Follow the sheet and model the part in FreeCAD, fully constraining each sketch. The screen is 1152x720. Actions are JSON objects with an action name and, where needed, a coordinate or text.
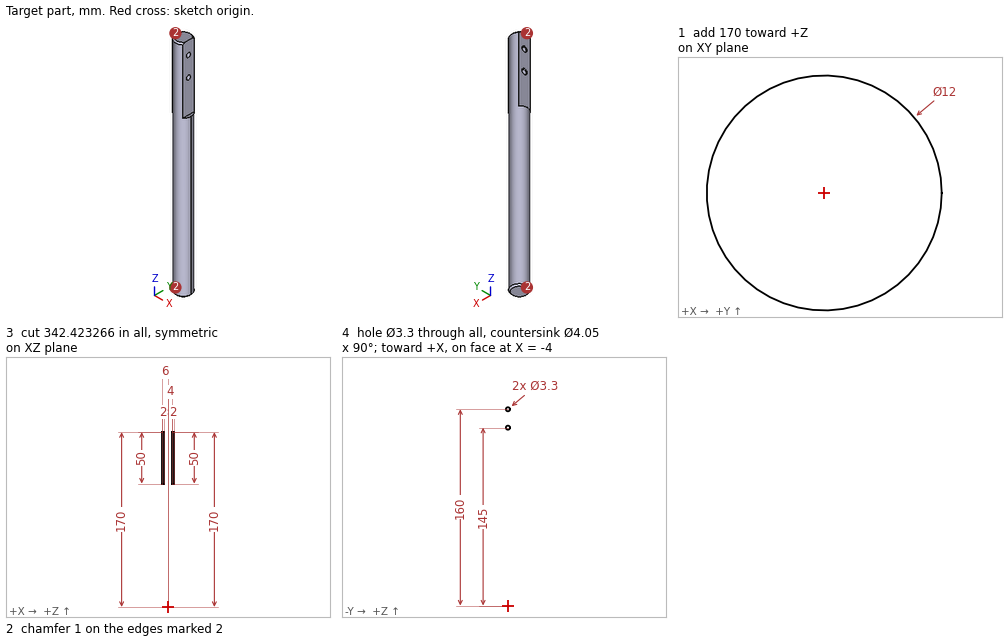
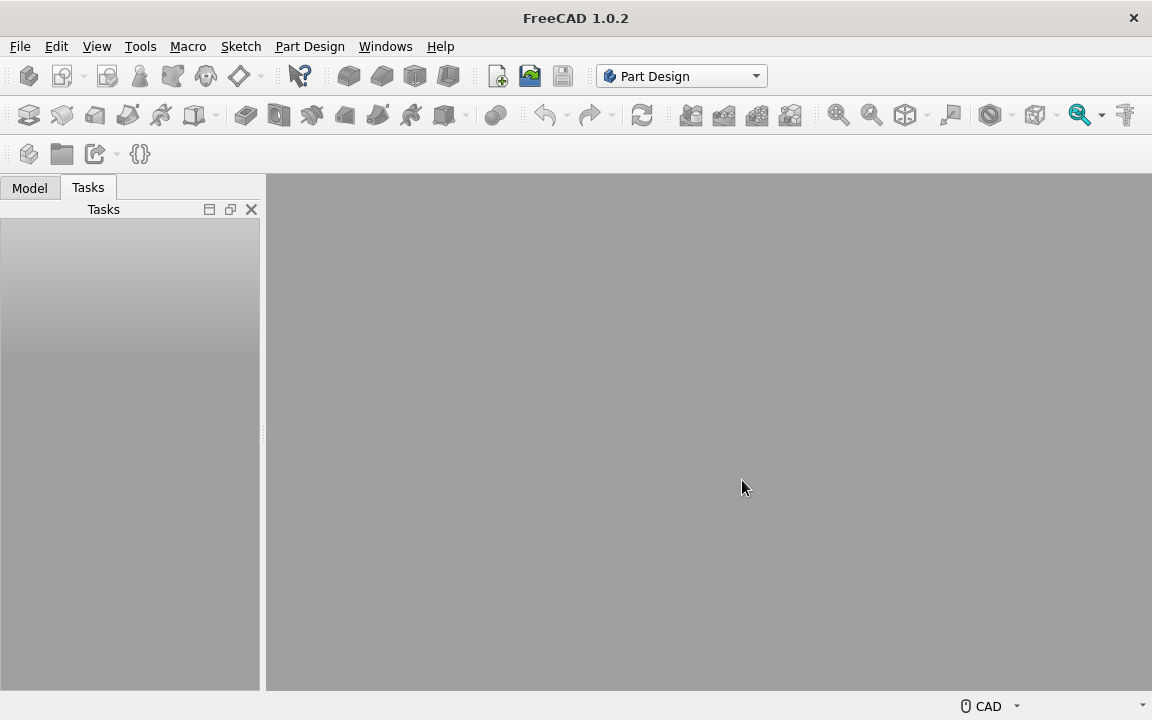
{"action": "key", "text": "ctrl+n"}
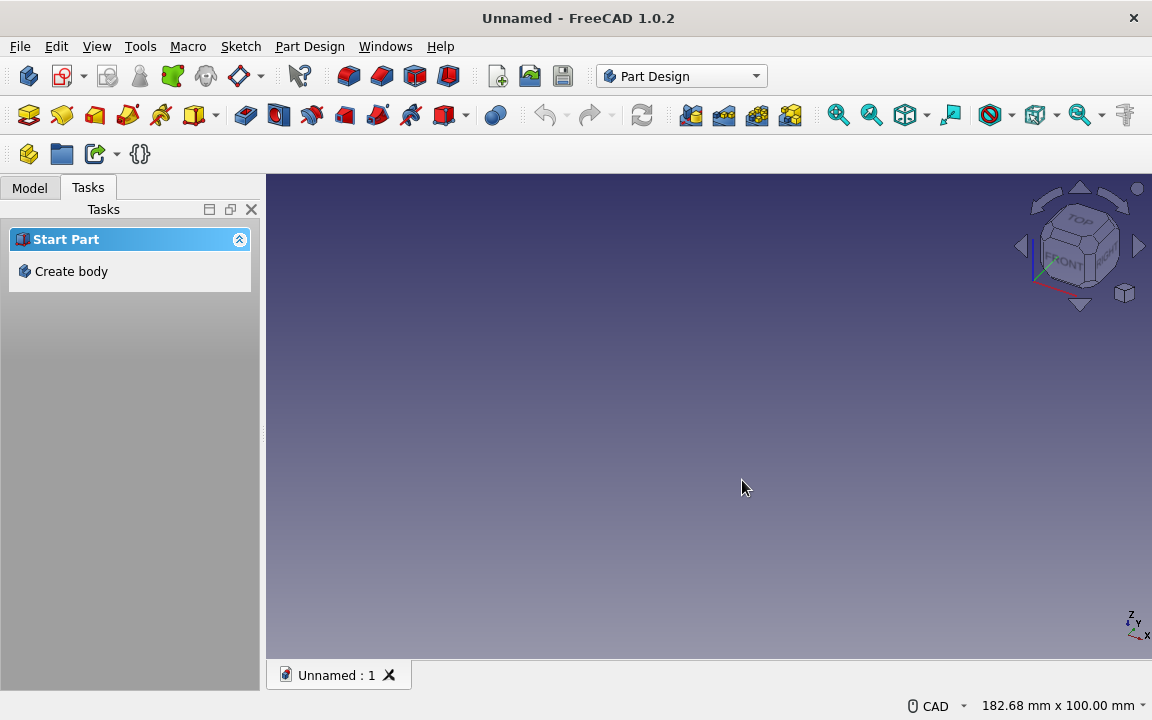
{"action": "left_click", "coordinate": [62, 76]}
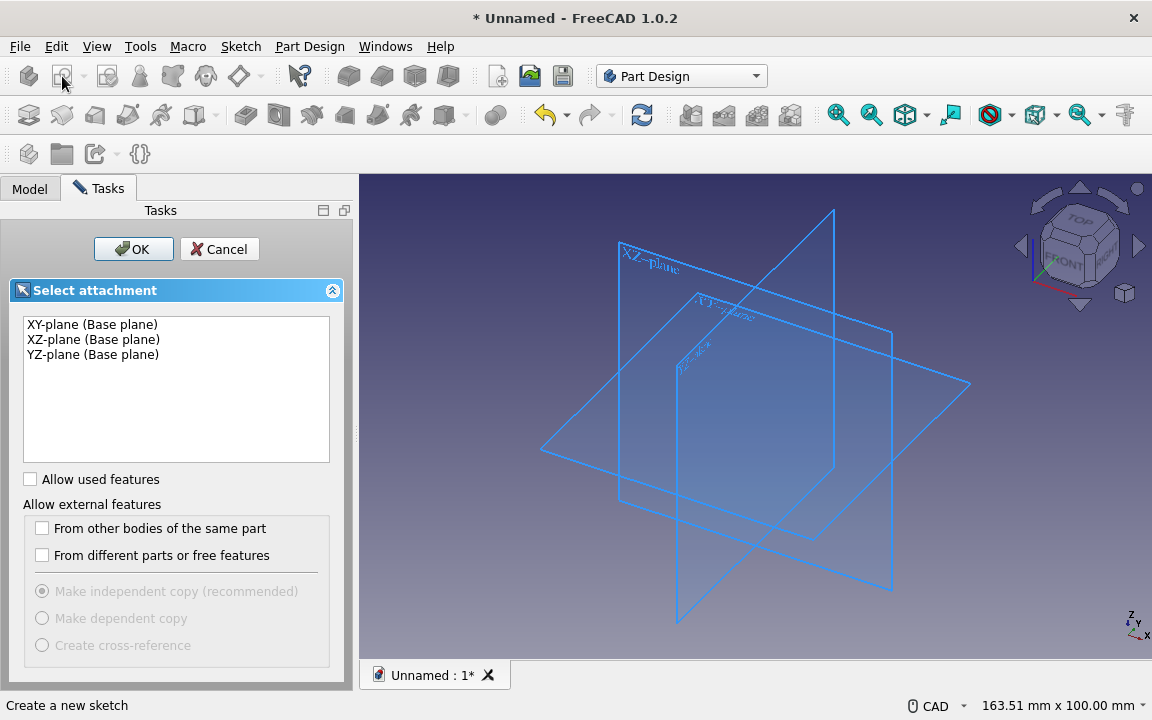
{"action": "left_click", "coordinate": [84, 324]}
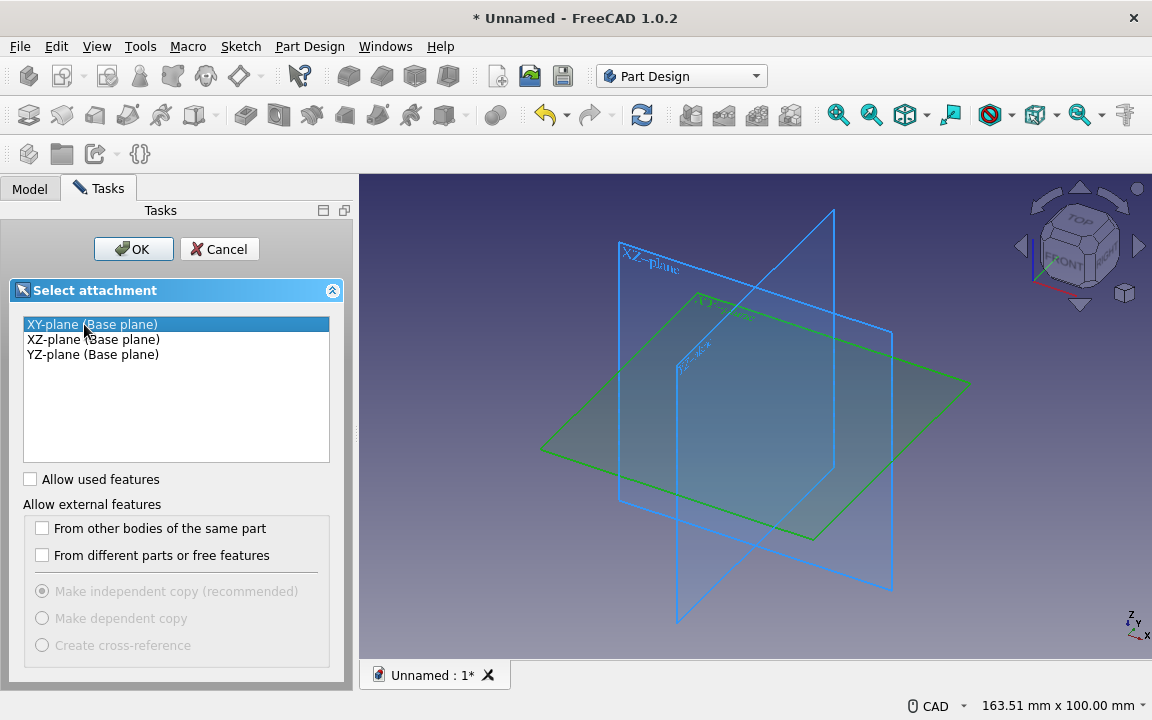
{"action": "left_click", "coordinate": [134, 249]}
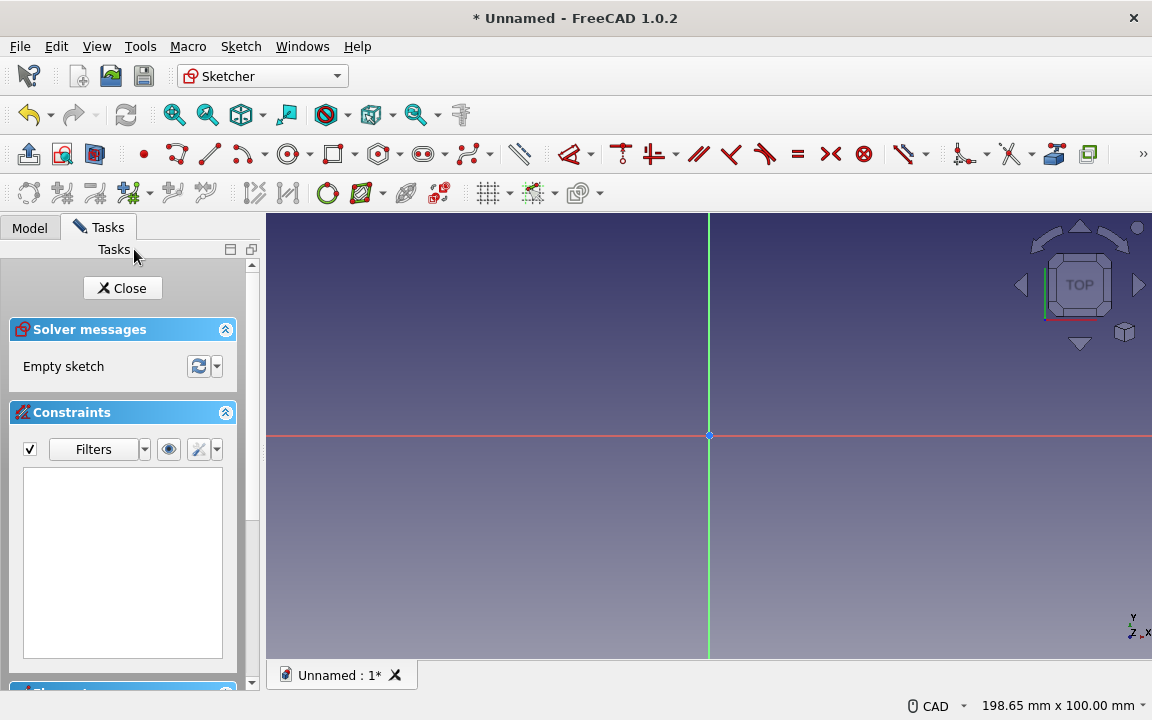
{"action": "scroll", "coordinate": [726, 436], "scroll_direction": "up", "scroll_amount": 8}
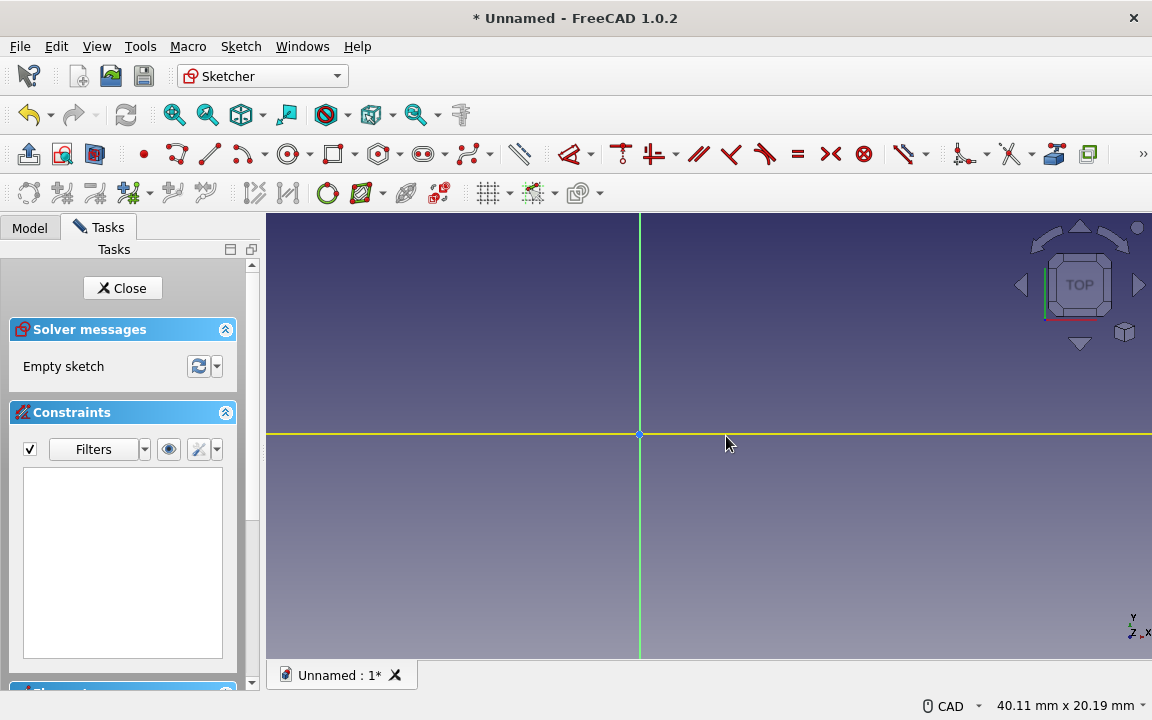
{"action": "key", "text": "g c"}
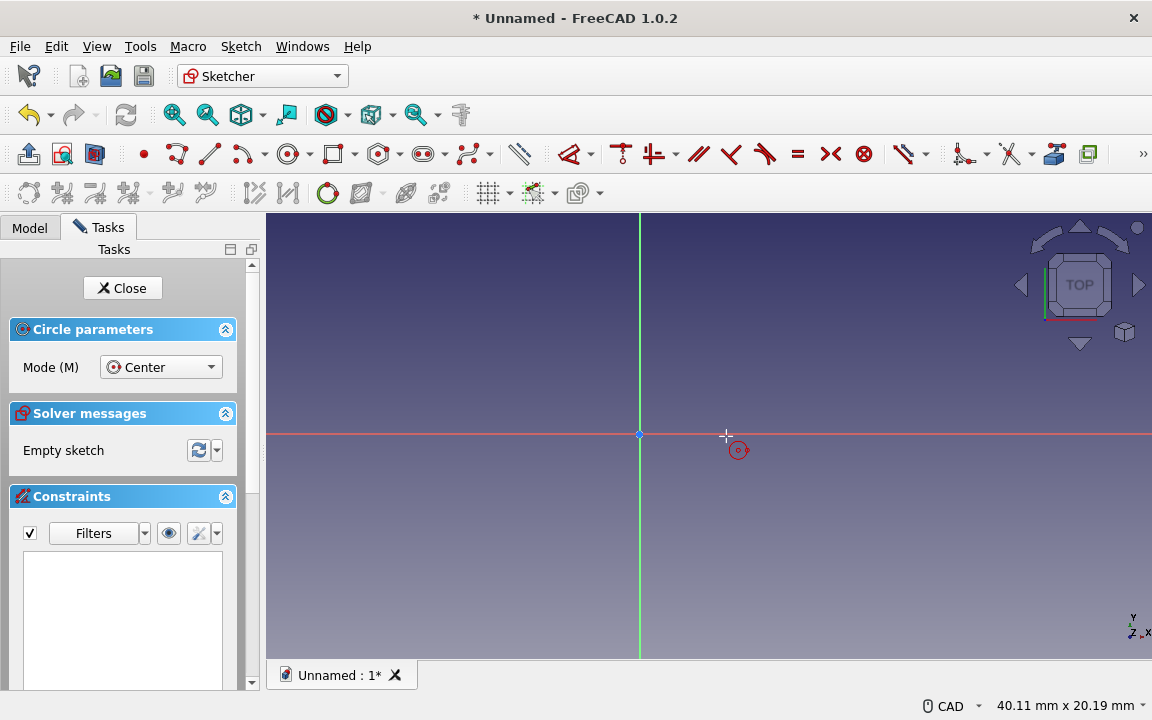
{"action": "left_click", "coordinate": [640, 434]}
{"action": "mouse_move", "coordinate": [733, 340]}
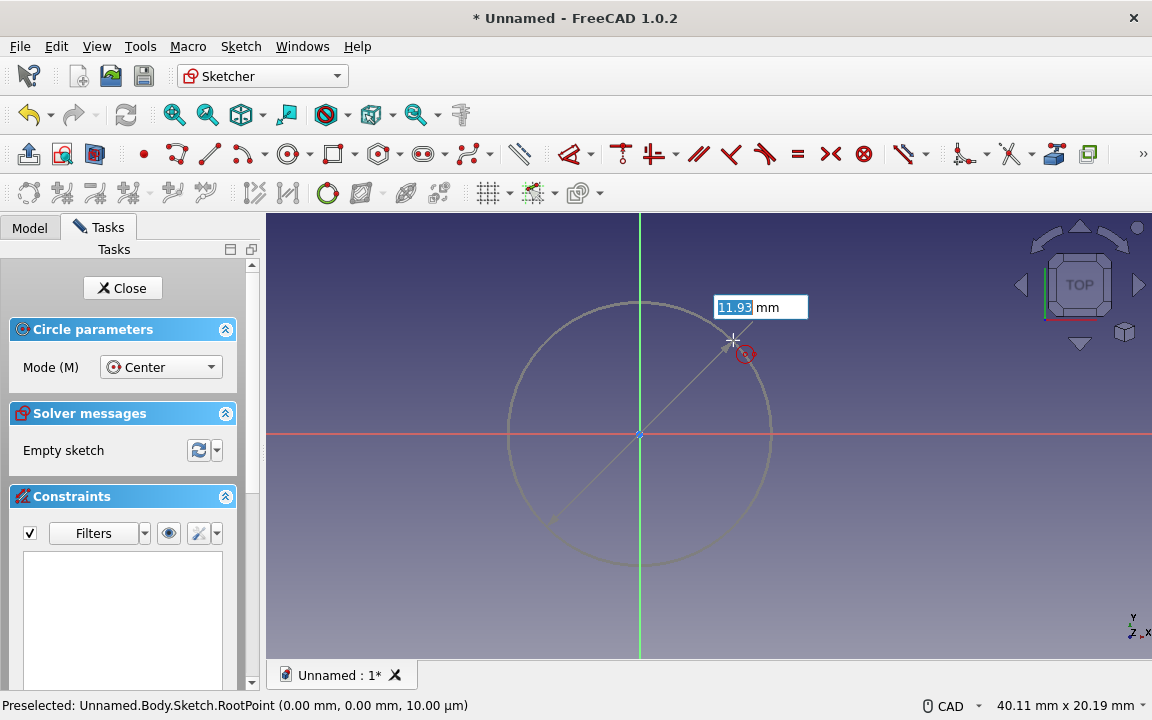
{"action": "type", "text": "12"}
{"action": "key", "text": "Return"}
{"action": "key", "text": "Escape"}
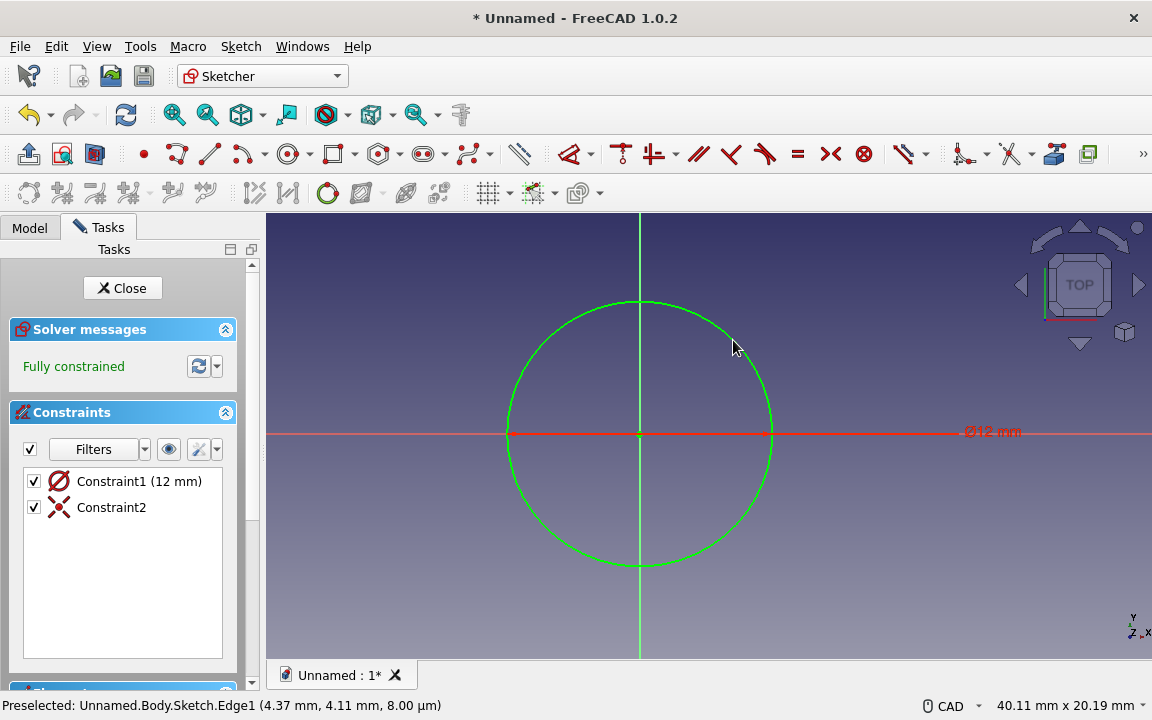
{"action": "left_click", "coordinate": [123, 288]}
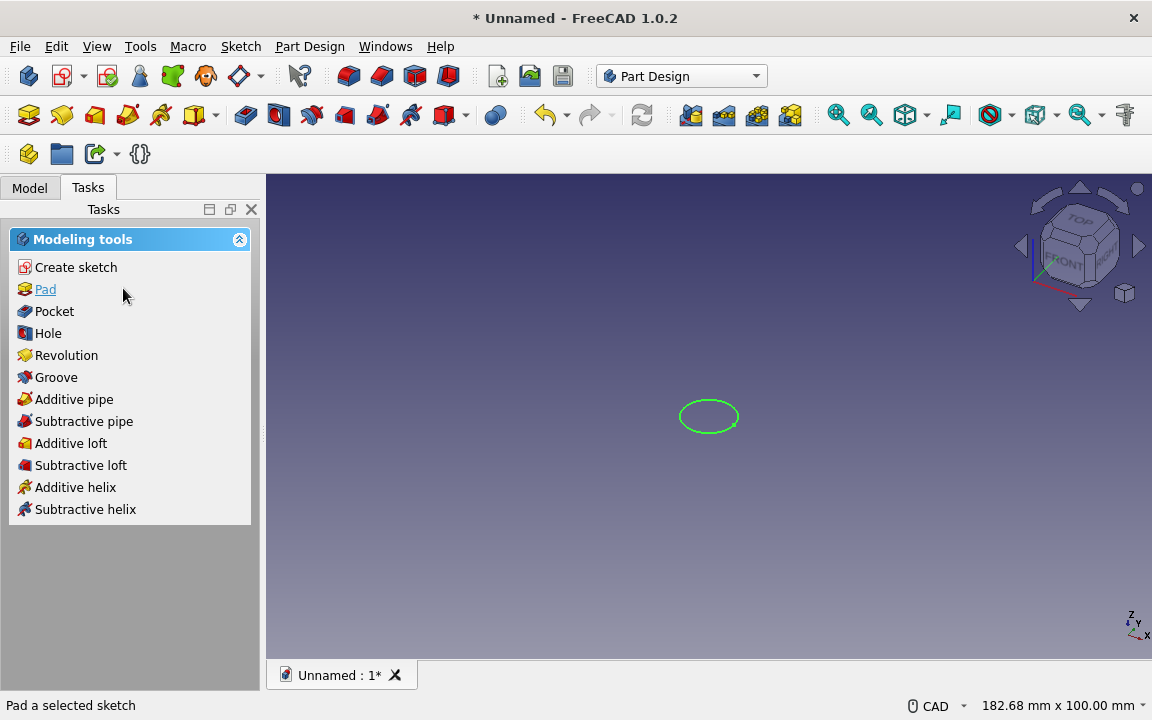
{"action": "left_click", "coordinate": [29, 116]}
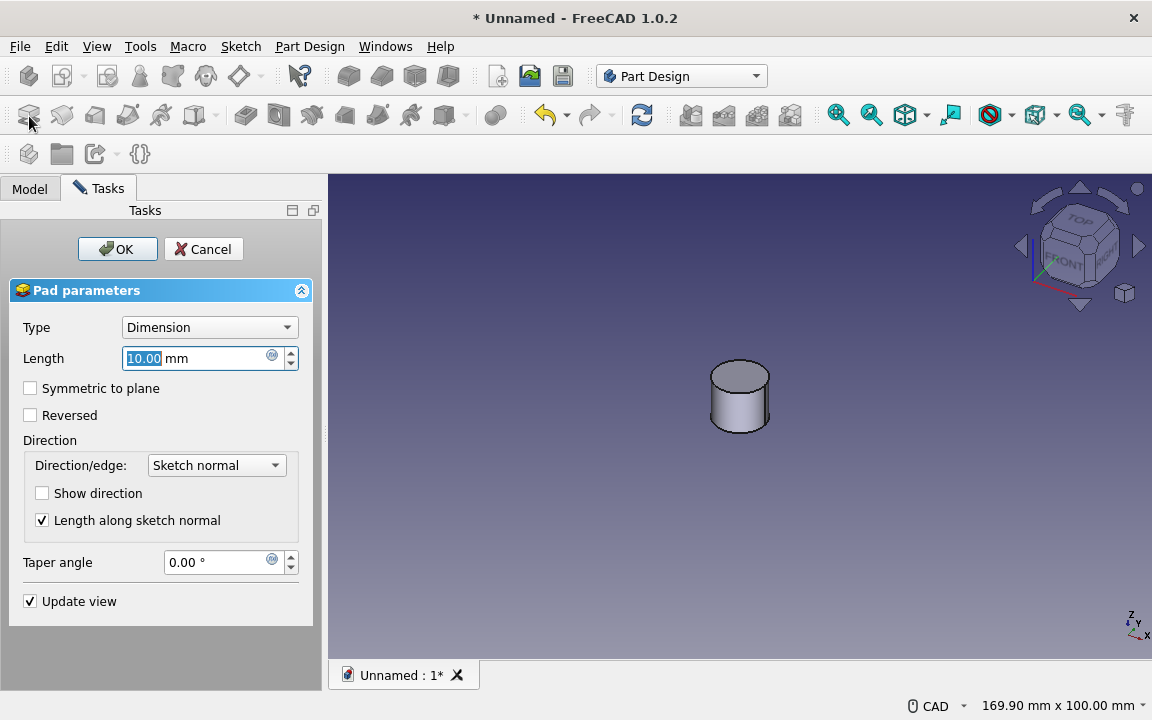
{"action": "type", "text": "170"}
{"action": "key", "text": "Tab"}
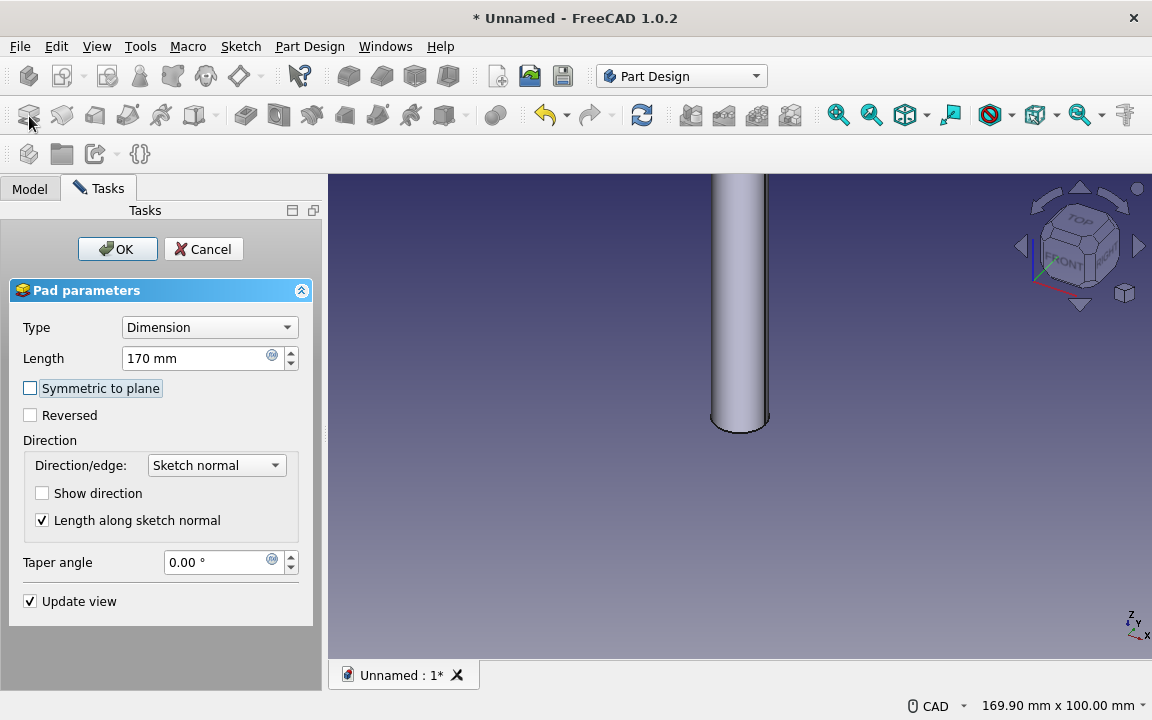
{"action": "left_click", "coordinate": [118, 249]}